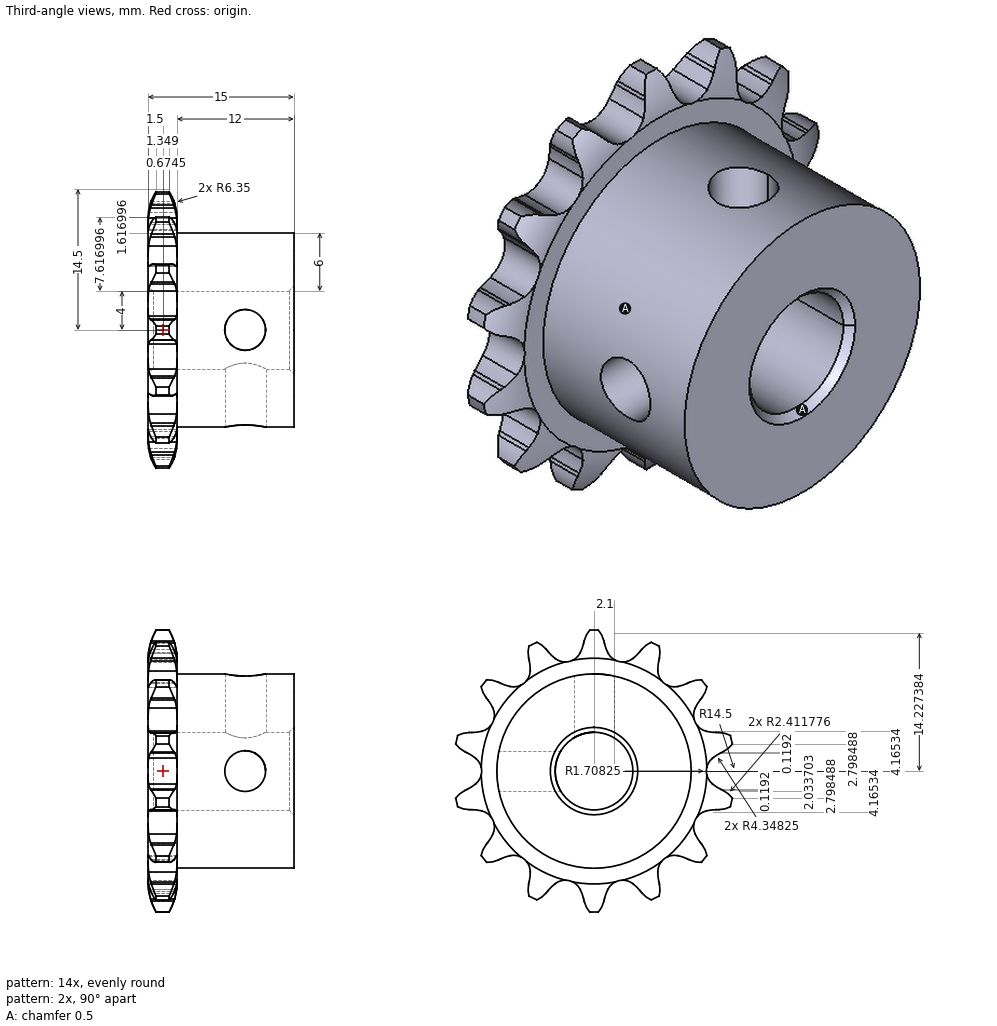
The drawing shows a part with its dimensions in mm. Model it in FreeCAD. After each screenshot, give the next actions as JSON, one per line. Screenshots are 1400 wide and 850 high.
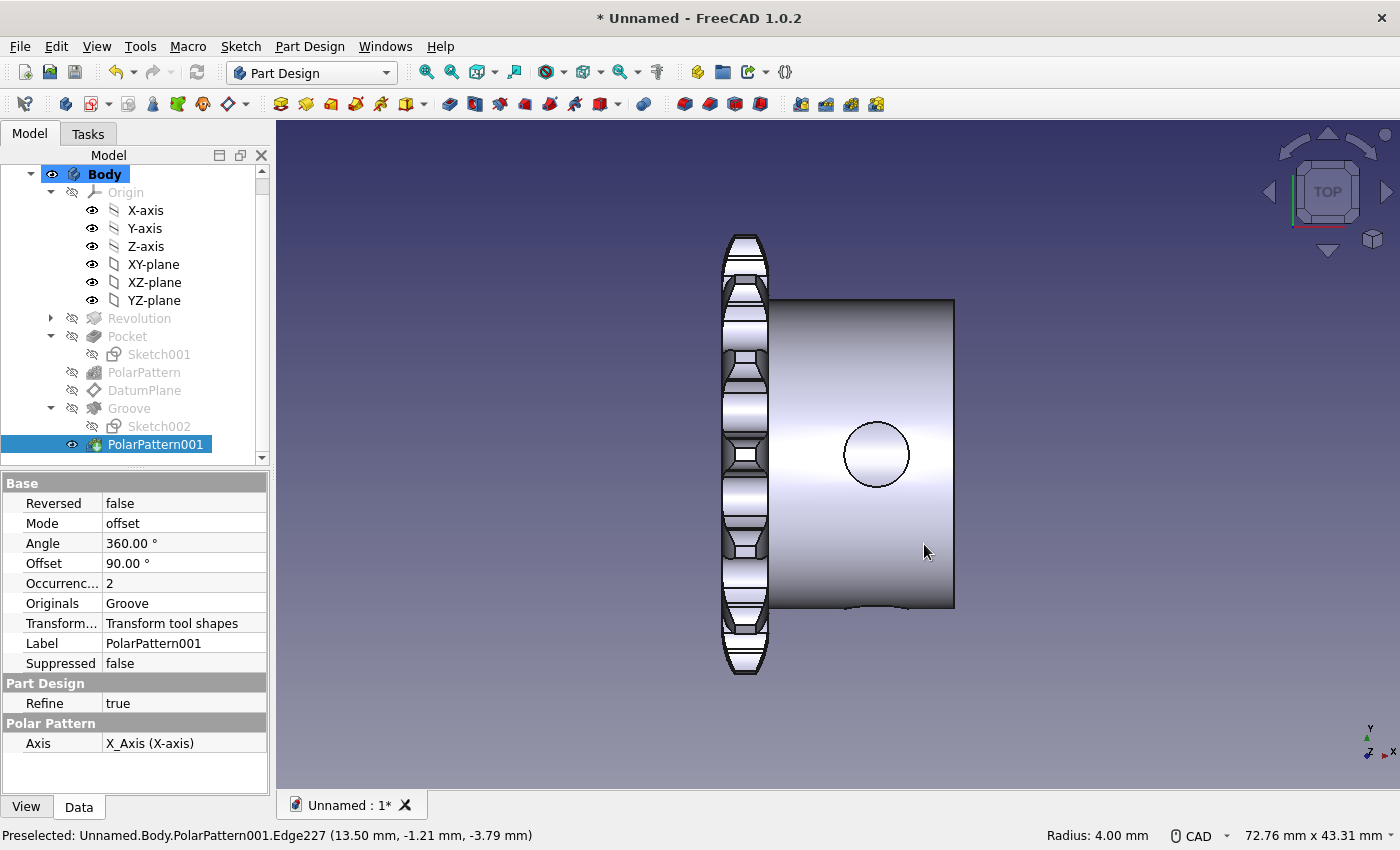
{"action": "key", "text": "1"}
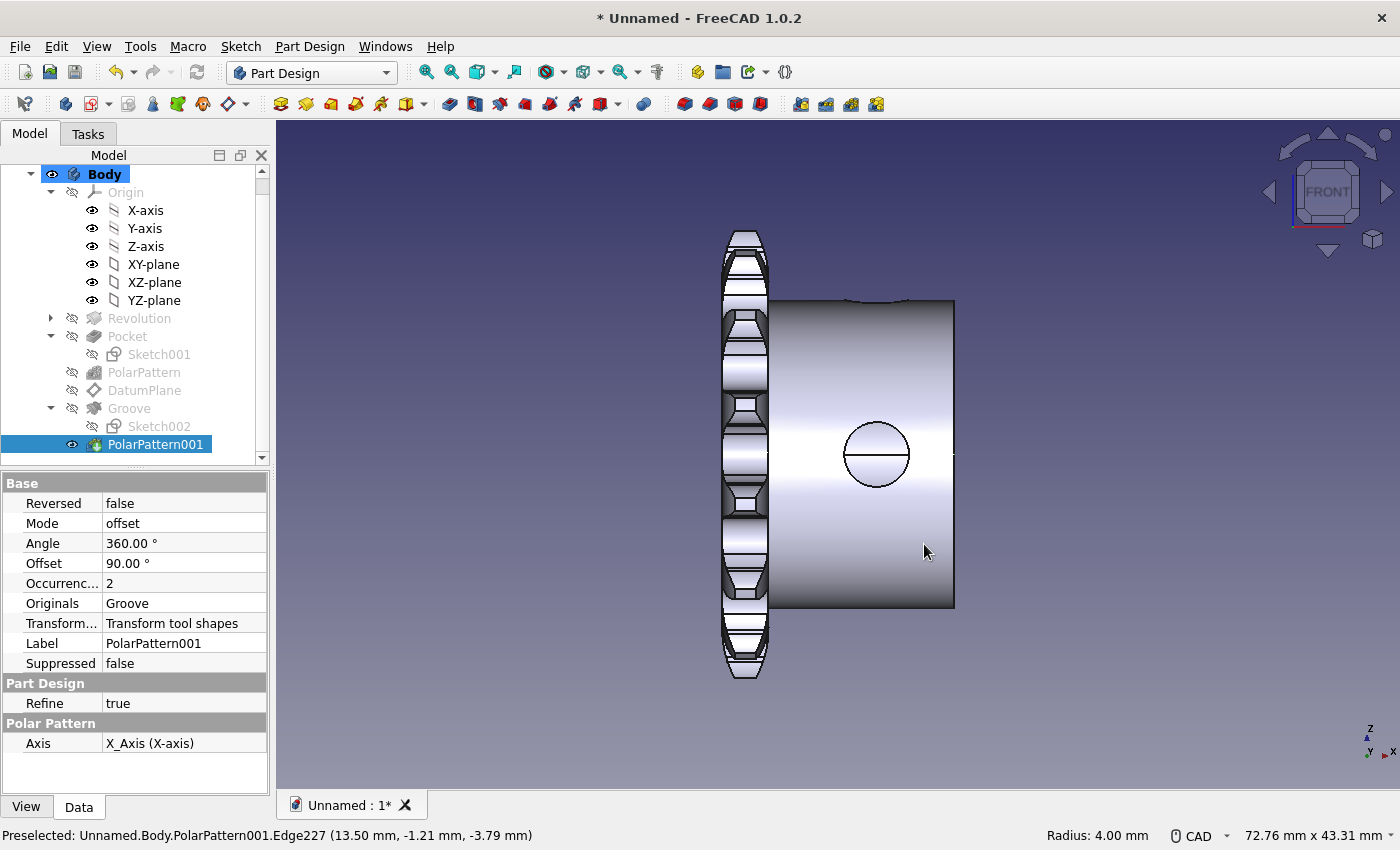
{"action": "key", "text": "3"}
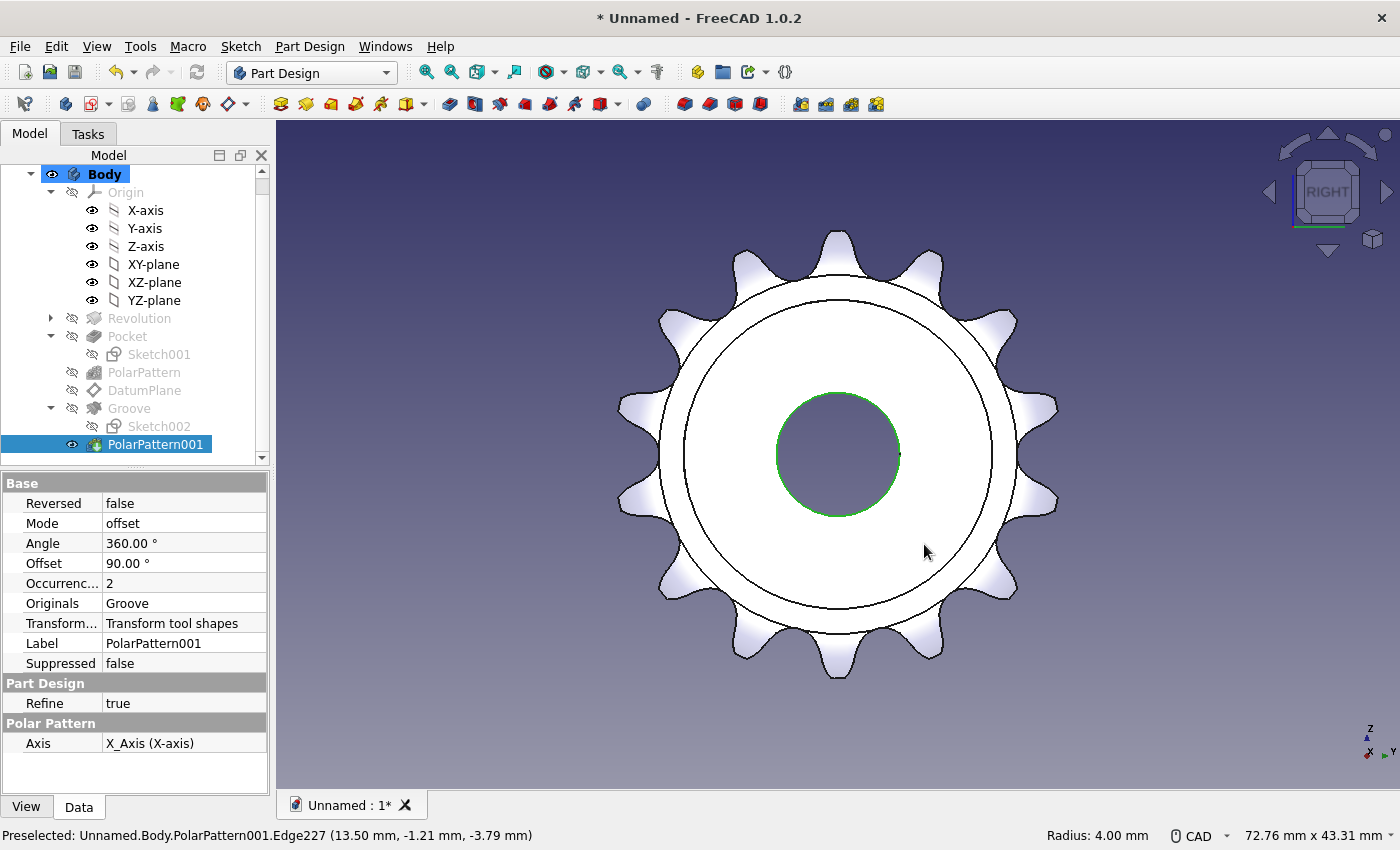
{"action": "key", "text": "5"}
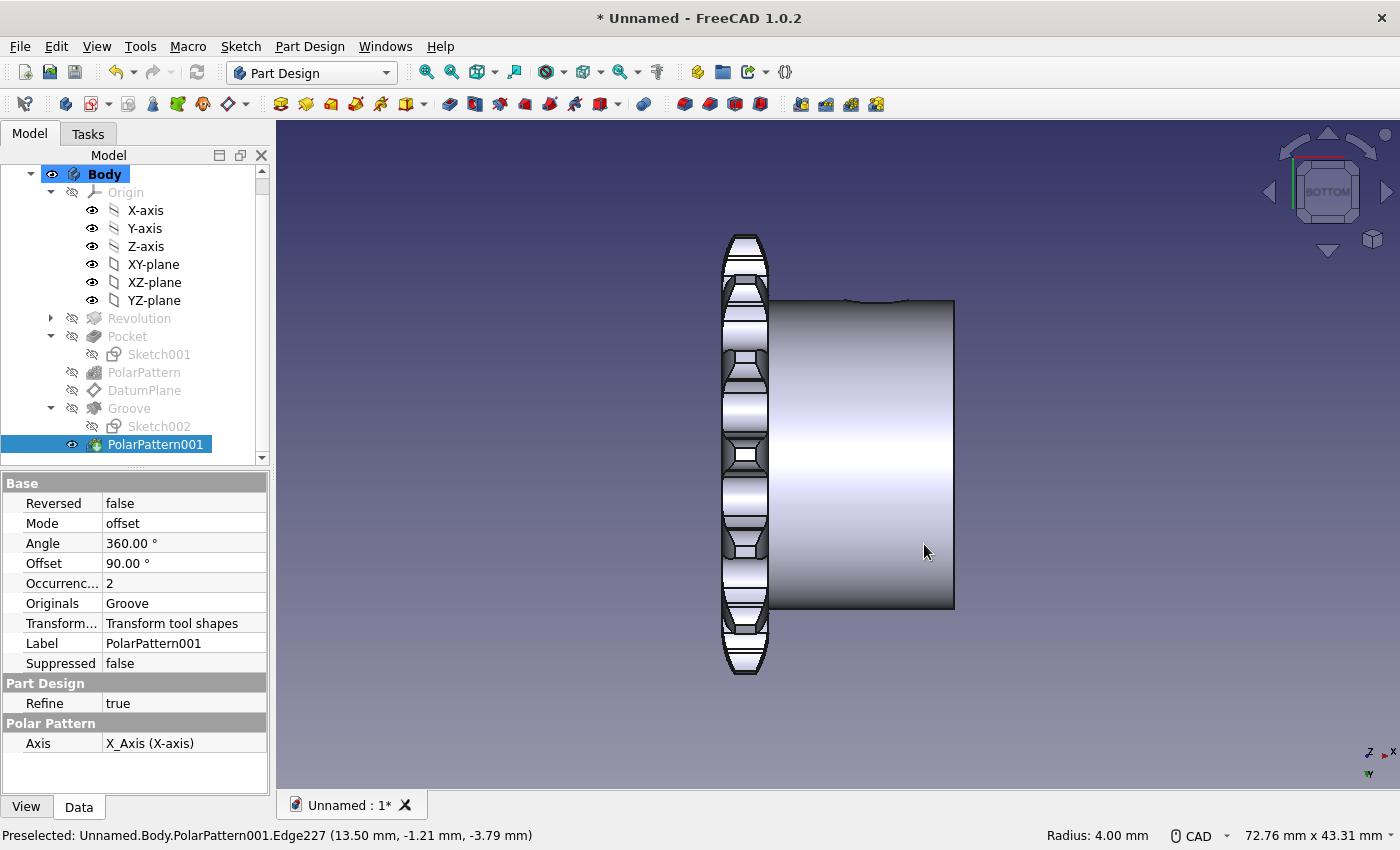
{"action": "key", "text": "4"}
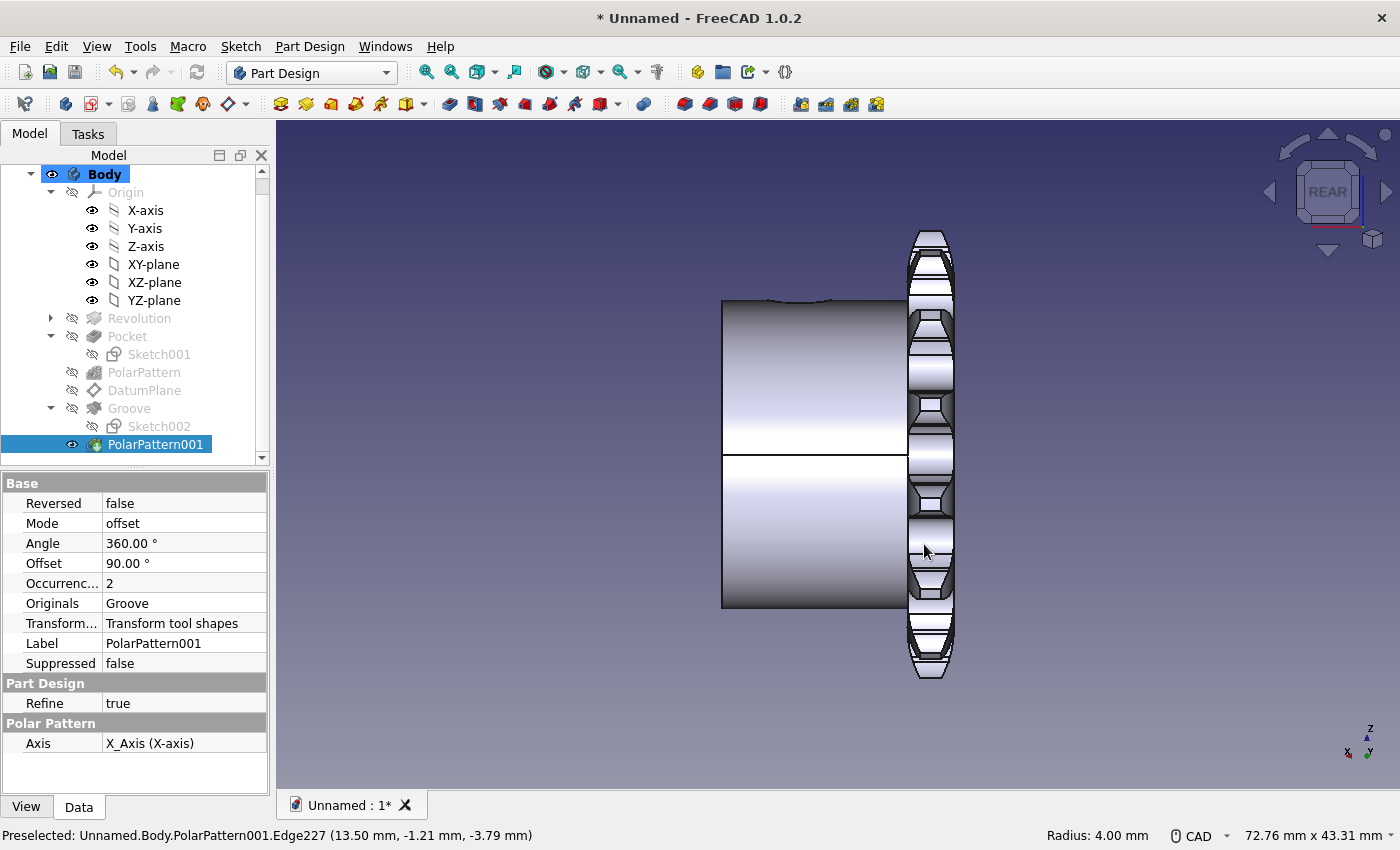
{"action": "key", "text": "6"}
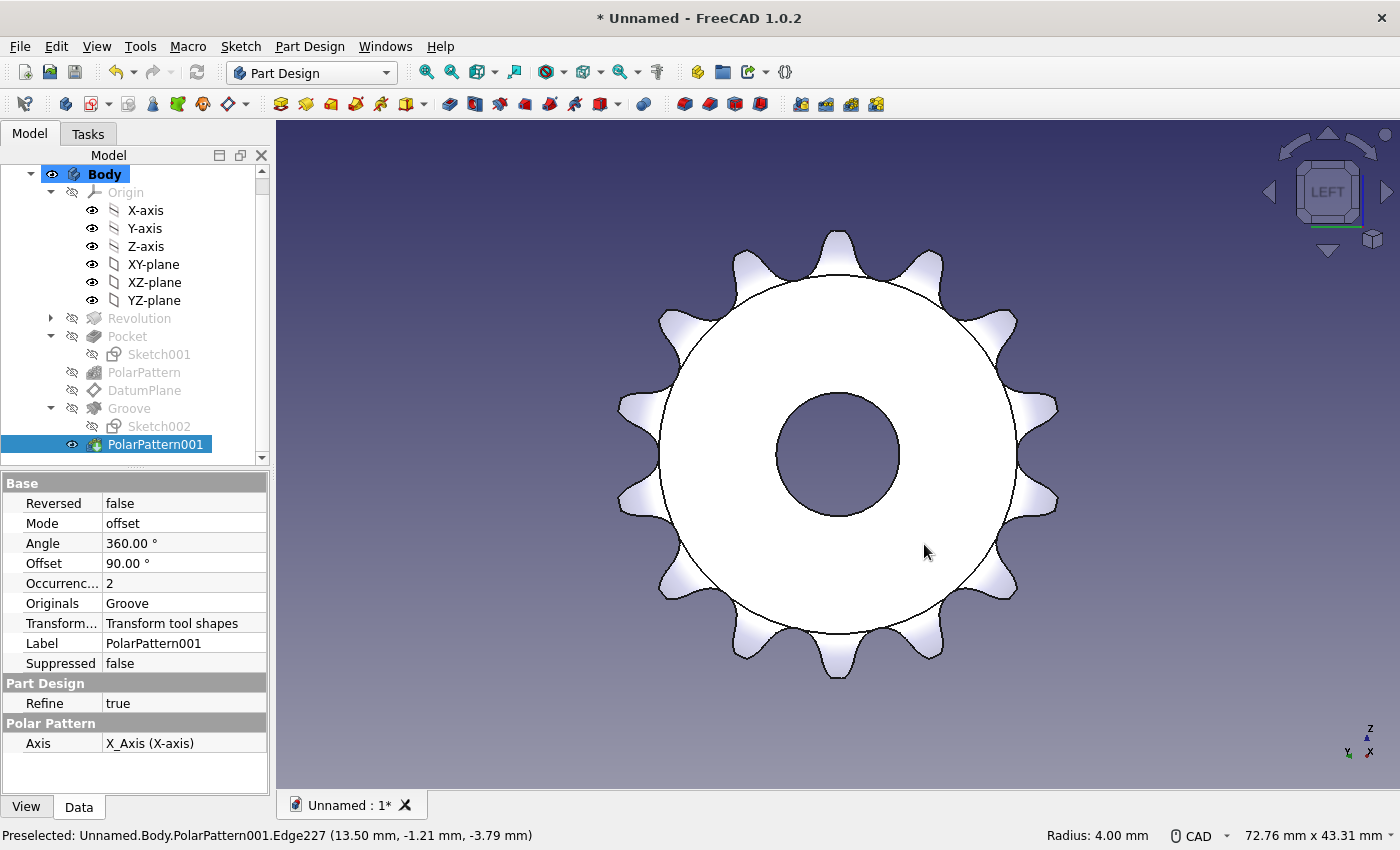
{"action": "left_click", "coordinate": [900, 453], "text": "ctrl"}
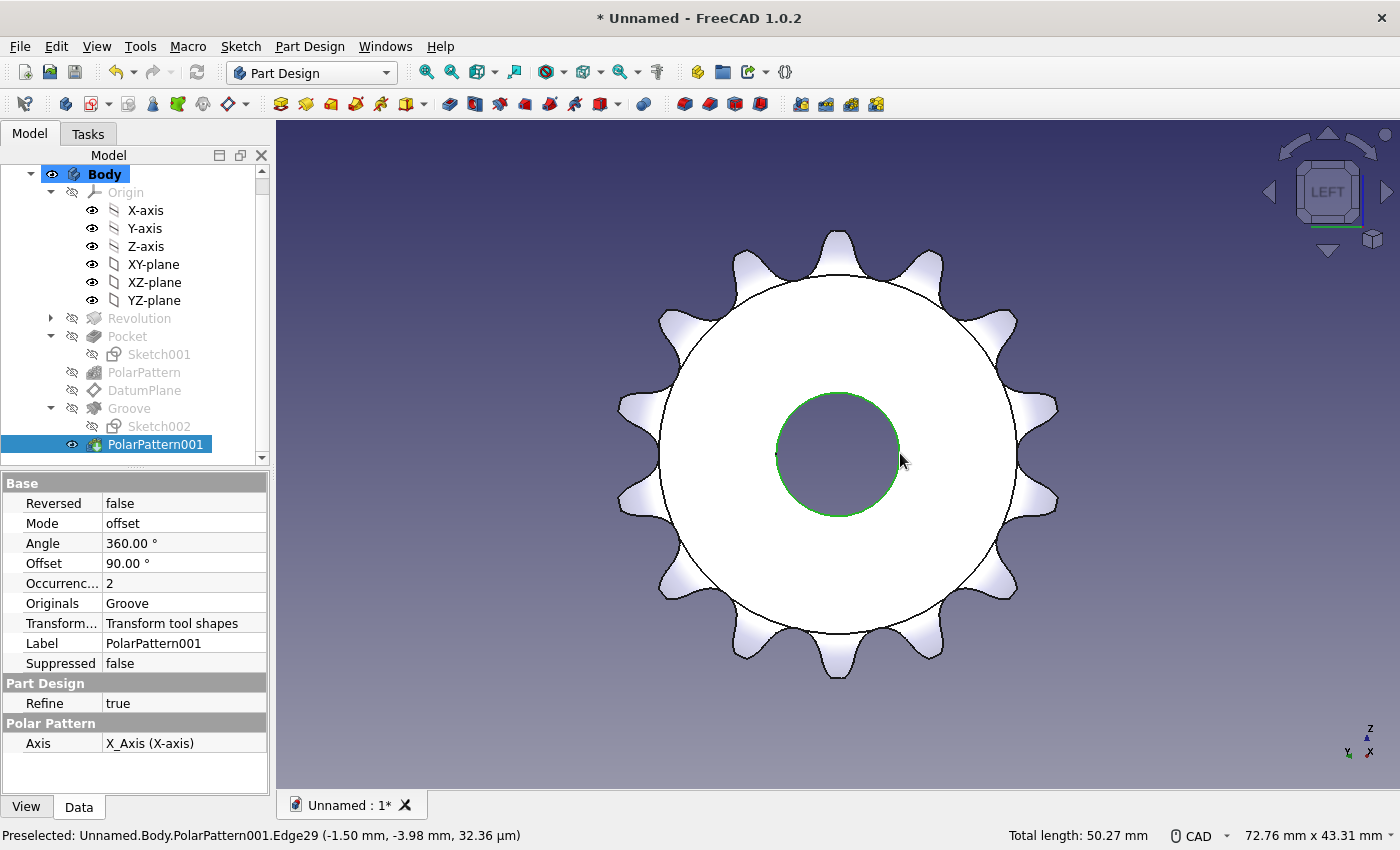
{"action": "left_click", "coordinate": [710, 104]}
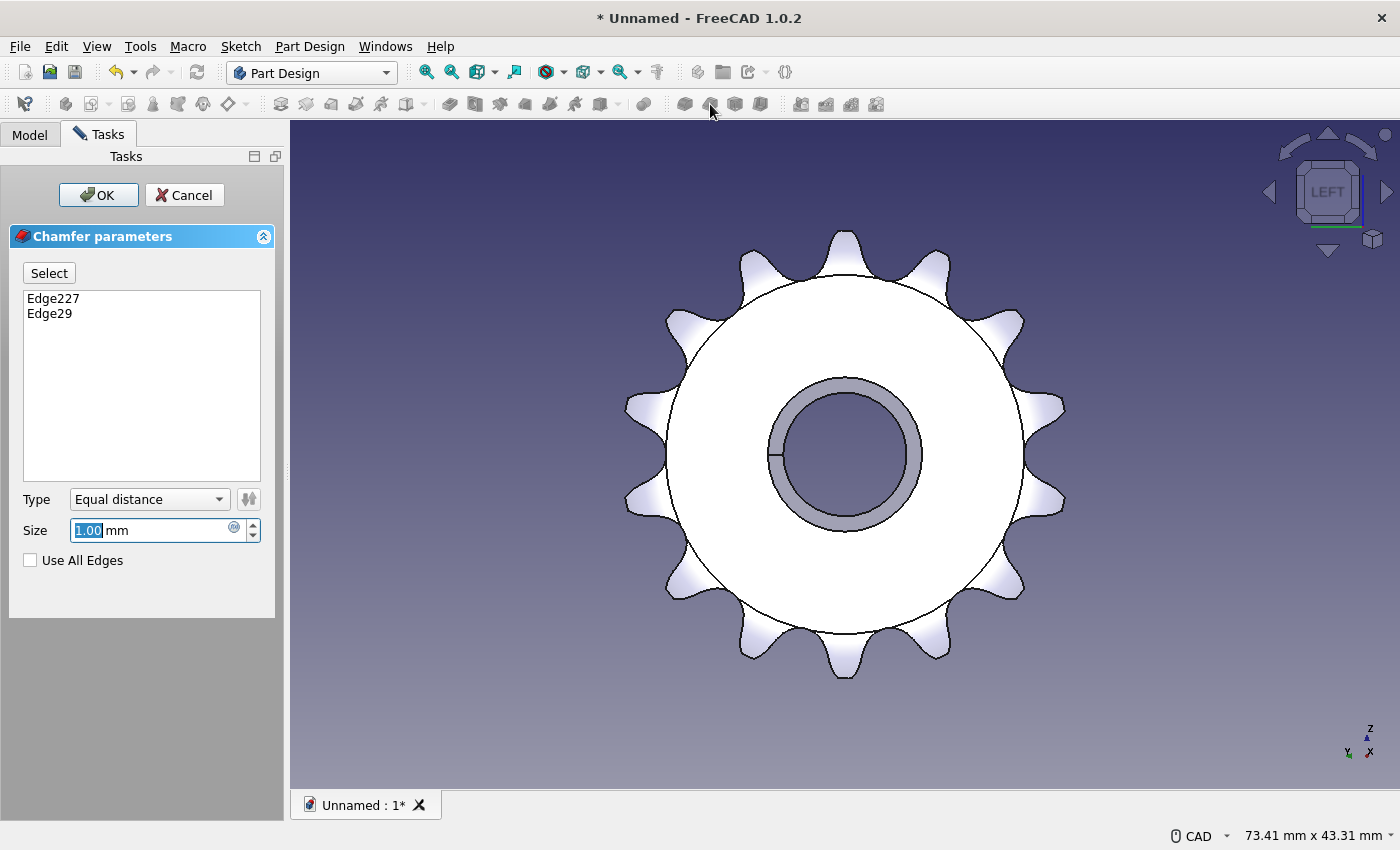
{"action": "type", "text": "0.5"}
{"action": "key", "text": "Tab"}